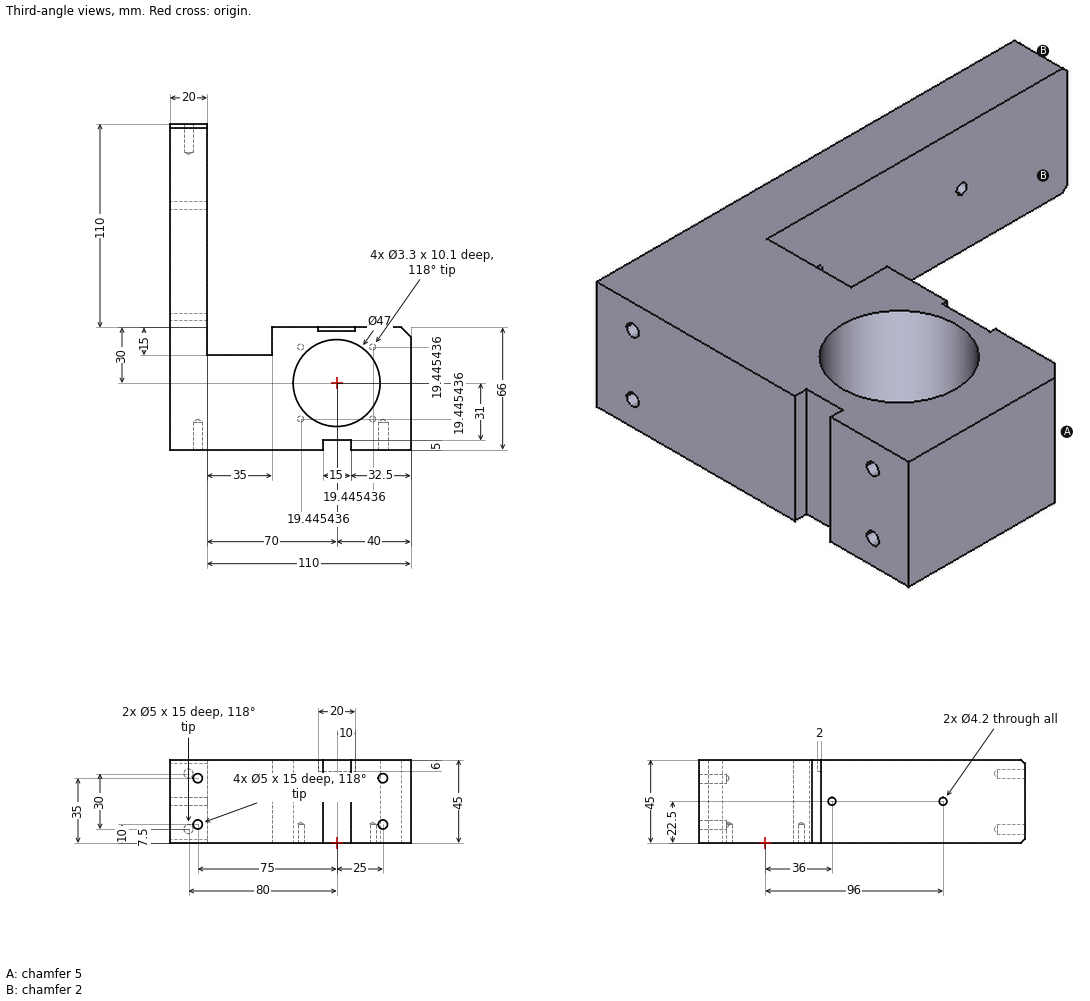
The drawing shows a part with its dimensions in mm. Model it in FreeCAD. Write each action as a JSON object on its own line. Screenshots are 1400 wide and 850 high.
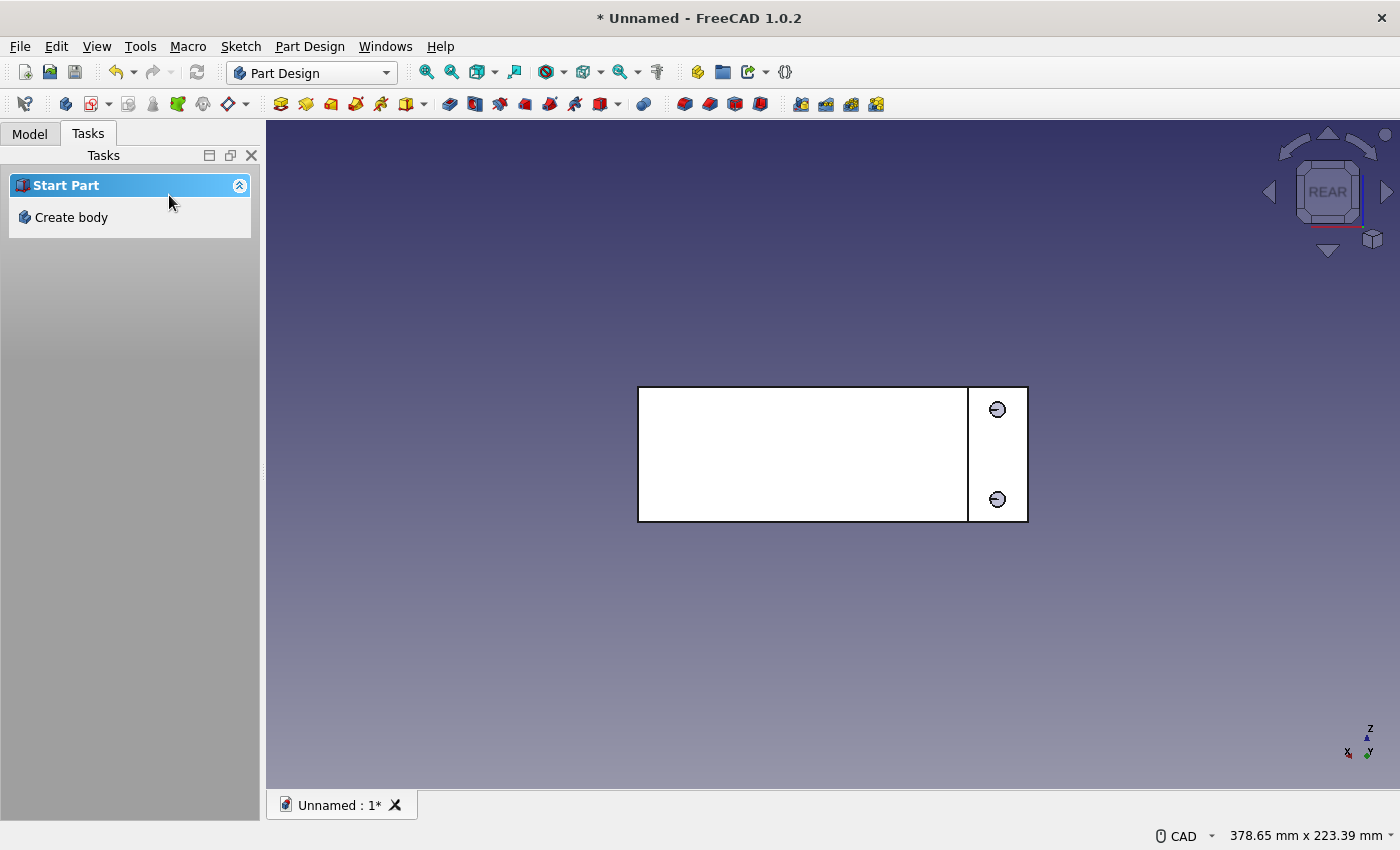
{"action": "left_click", "coordinate": [427, 72]}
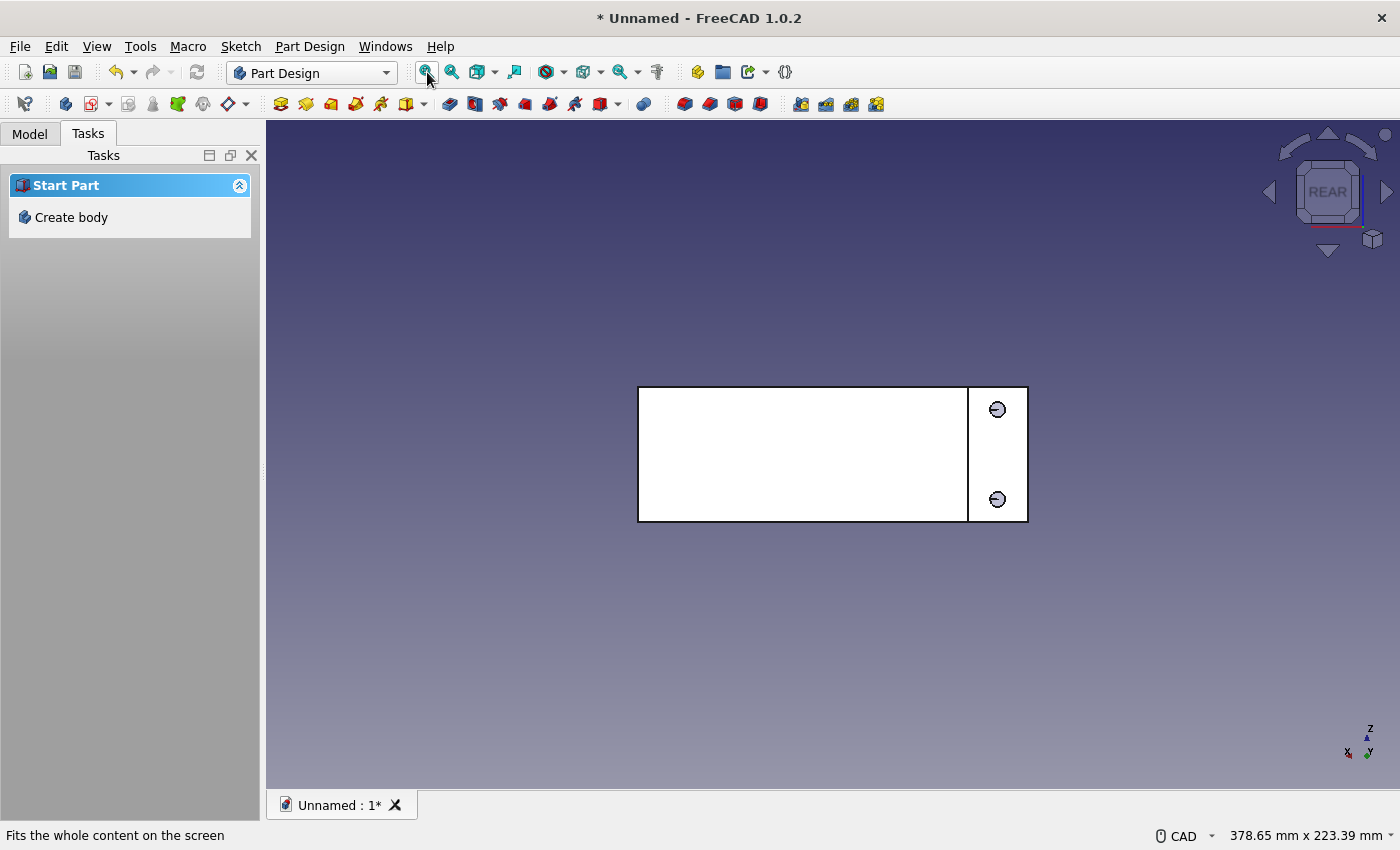
{"action": "left_click", "coordinate": [90, 104]}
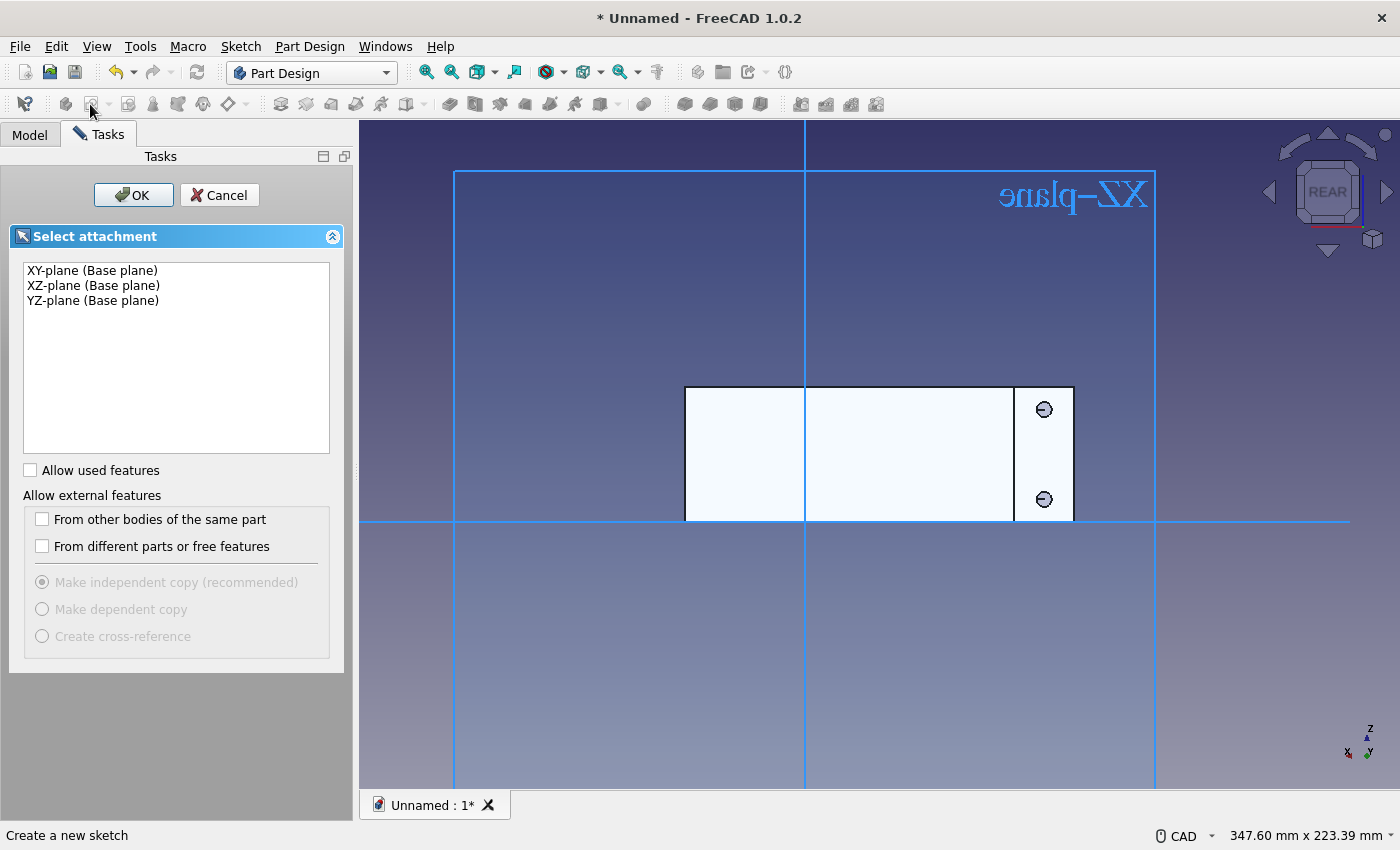
{"action": "left_click", "coordinate": [84, 270]}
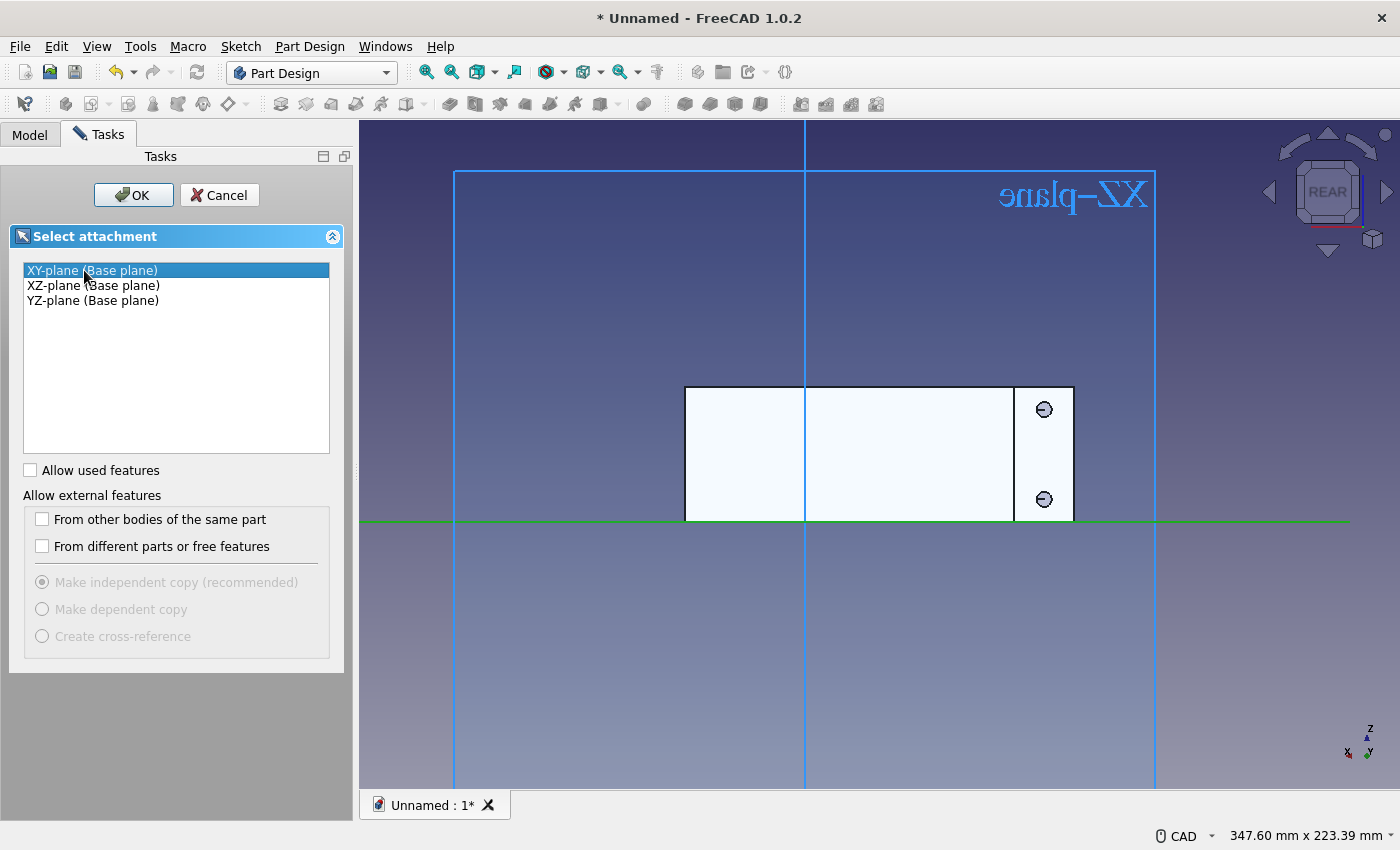
{"action": "left_click", "coordinate": [134, 195]}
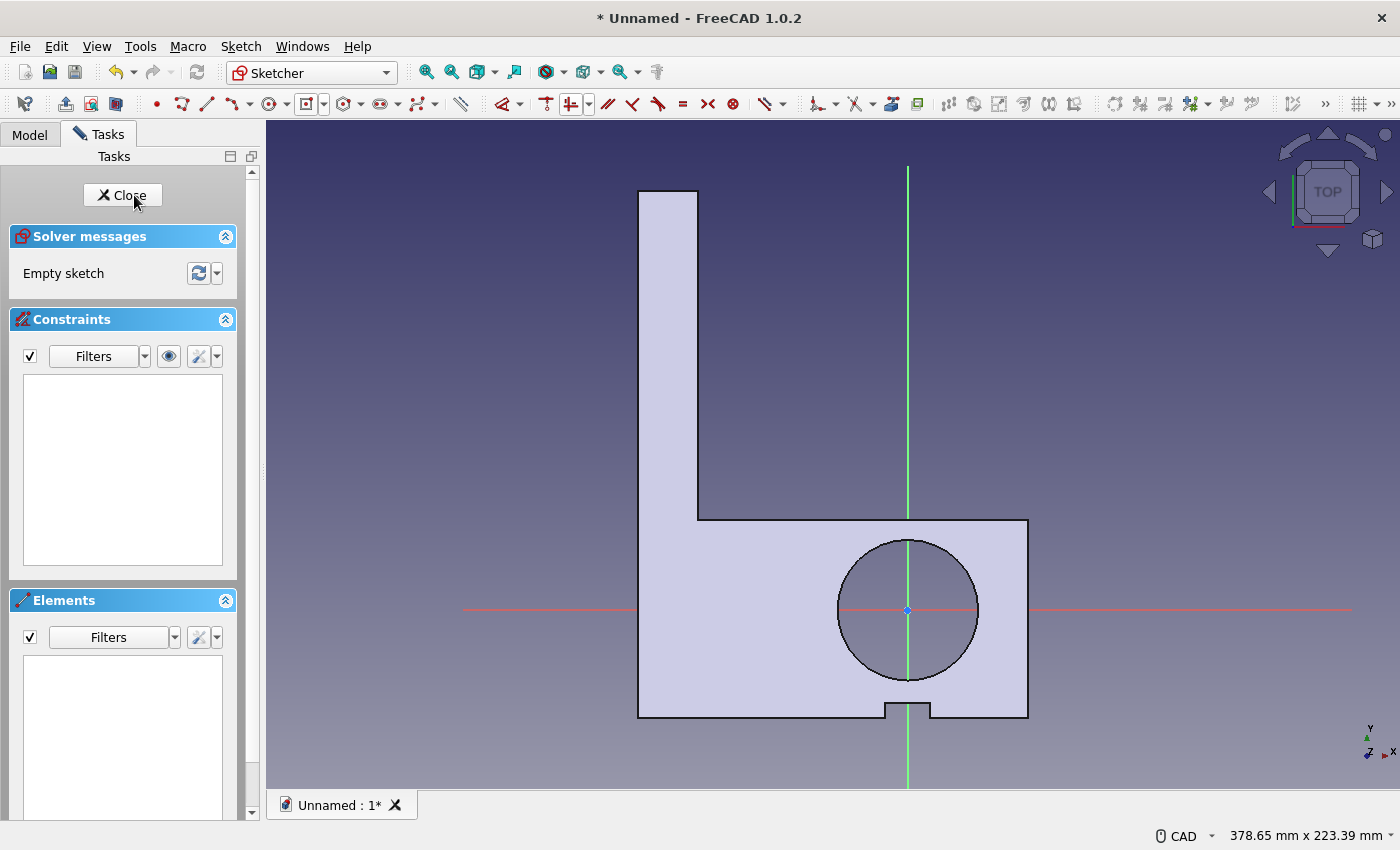
{"action": "key", "text": "q s"}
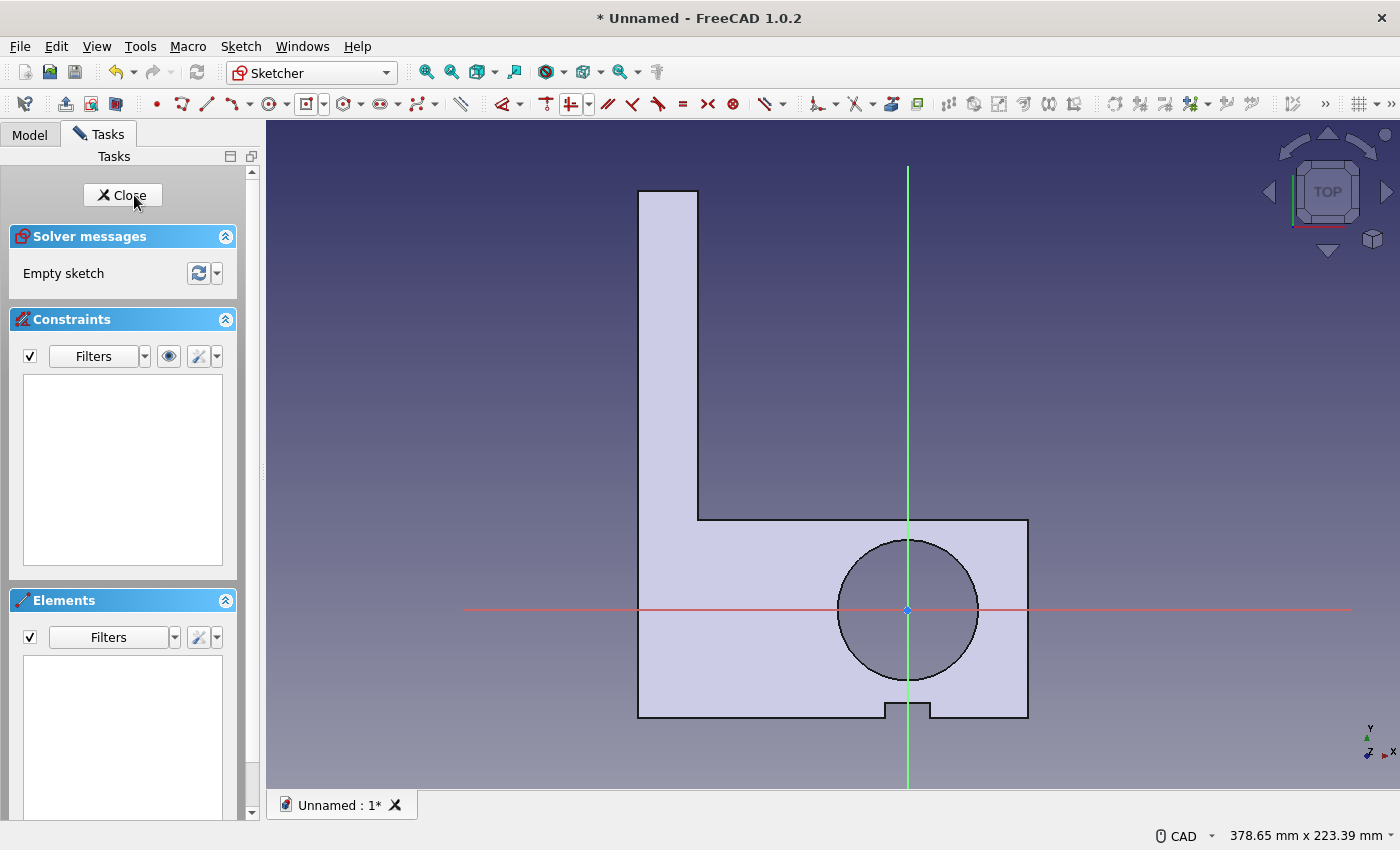
{"action": "scroll", "coordinate": [970, 677], "scroll_direction": "up", "scroll_amount": 6}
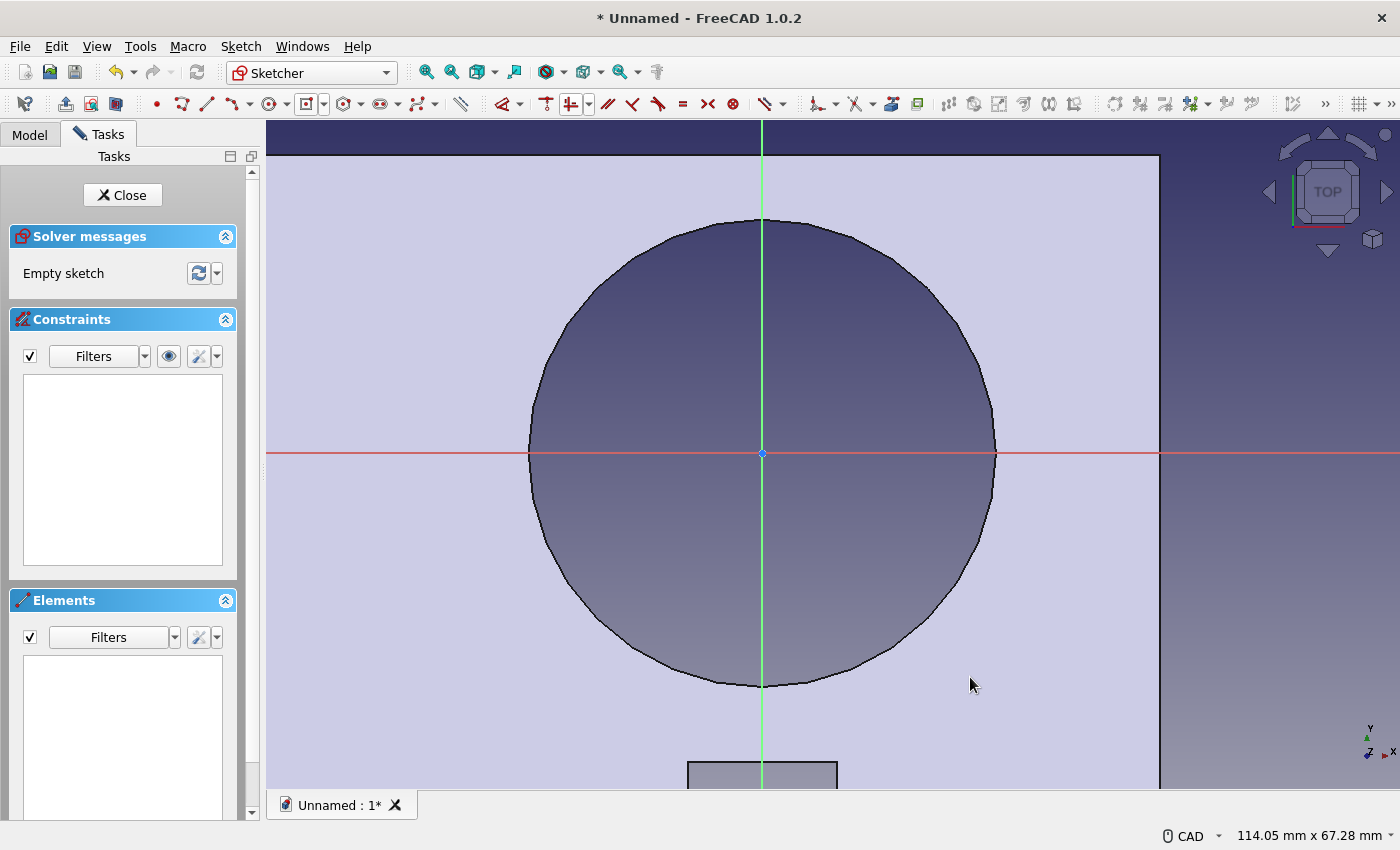
{"action": "left_click", "coordinate": [268, 104]}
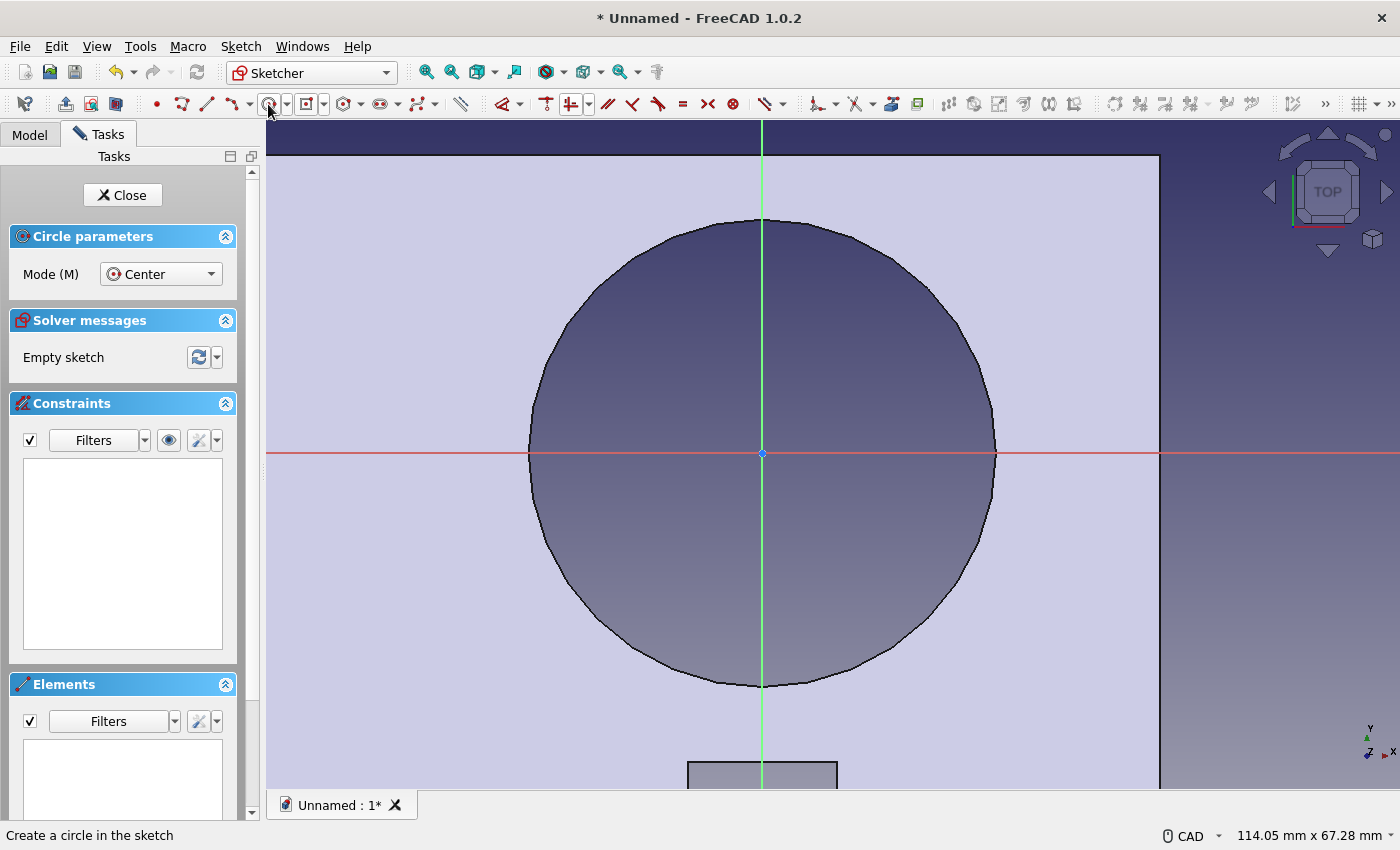
{"action": "scroll", "coordinate": [956, 260], "scroll_direction": "up", "scroll_amount": 2}